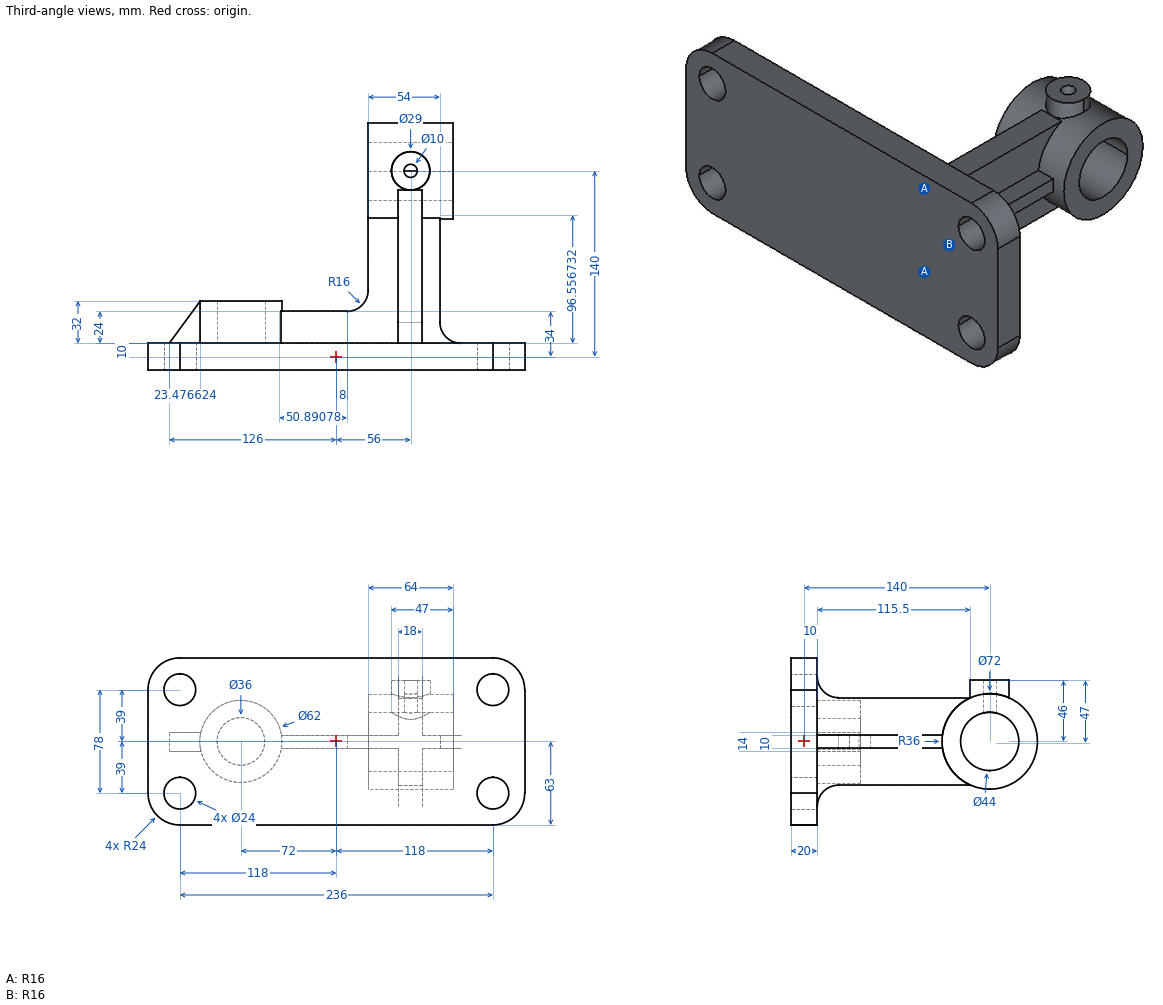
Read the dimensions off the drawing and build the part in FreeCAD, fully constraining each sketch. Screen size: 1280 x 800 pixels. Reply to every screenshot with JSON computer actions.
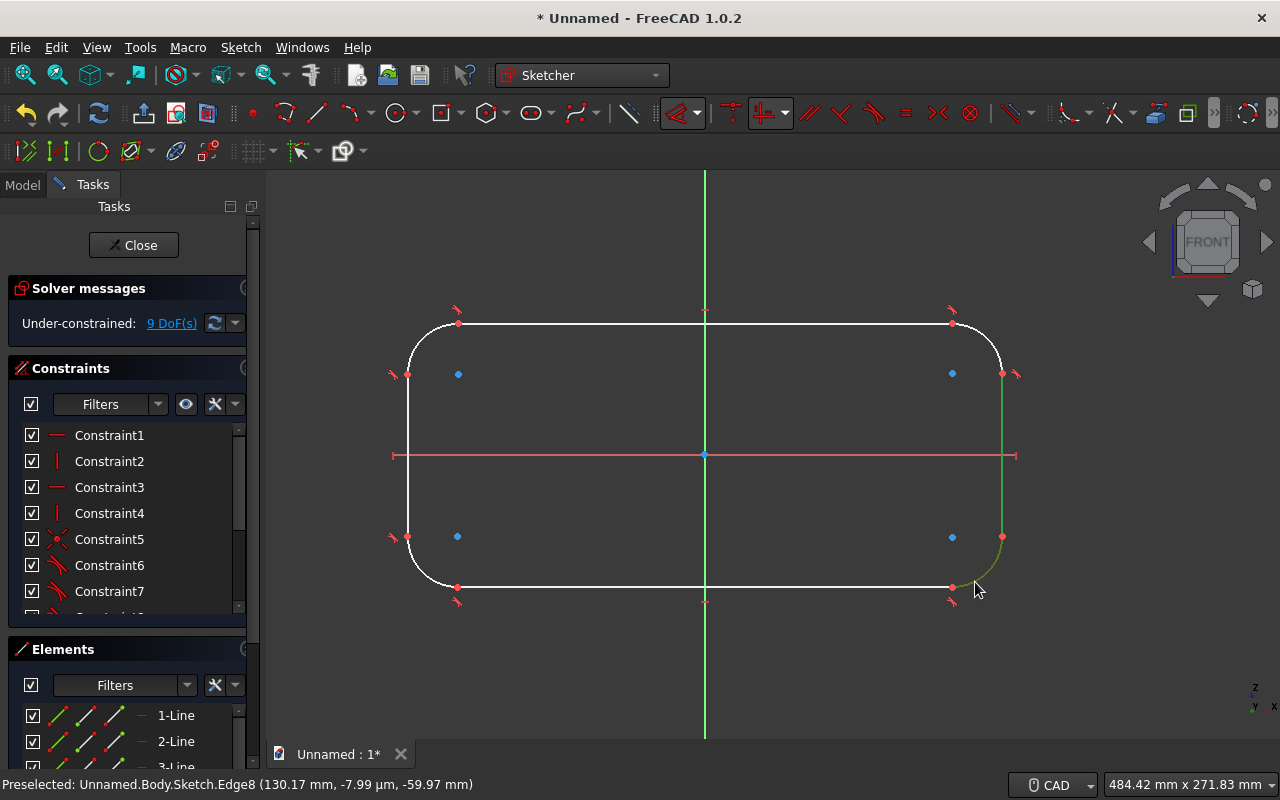
{"action": "left_click", "coordinate": [874, 114]}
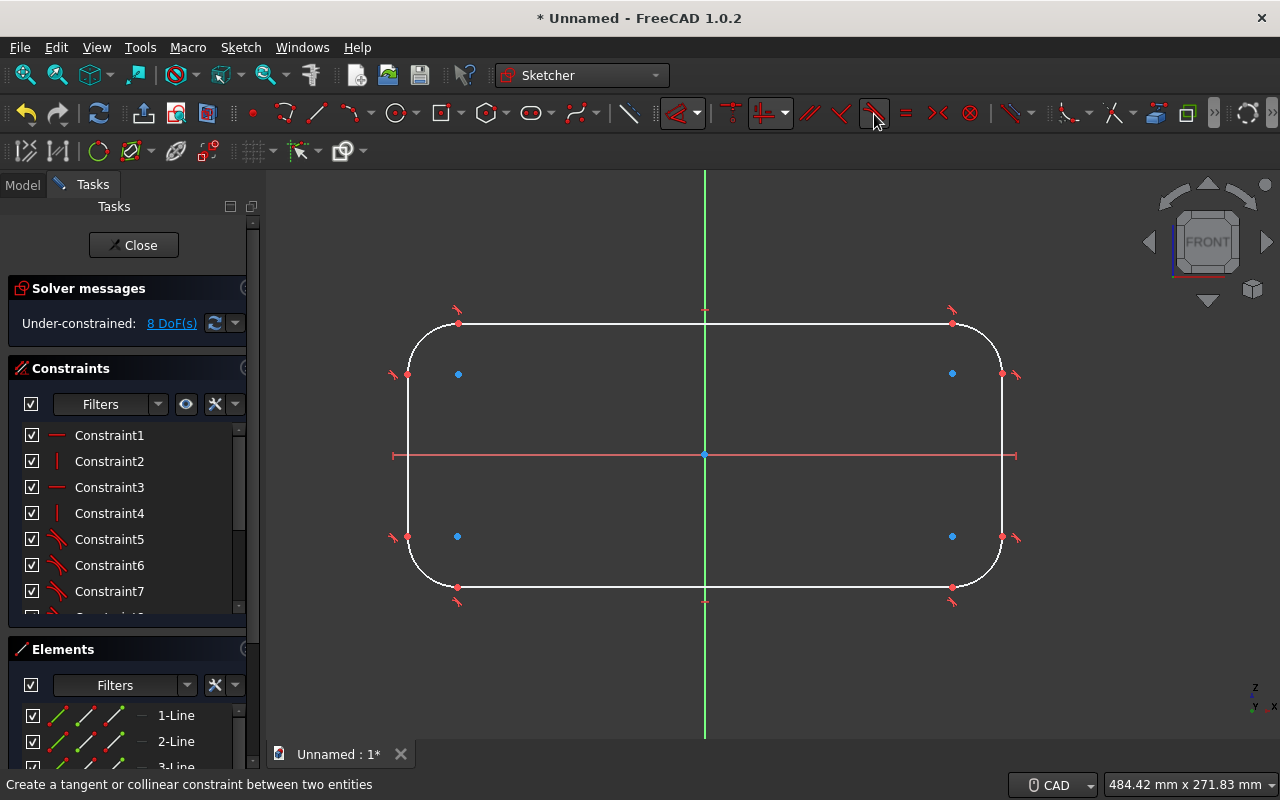
{"action": "left_click", "coordinate": [413, 560]}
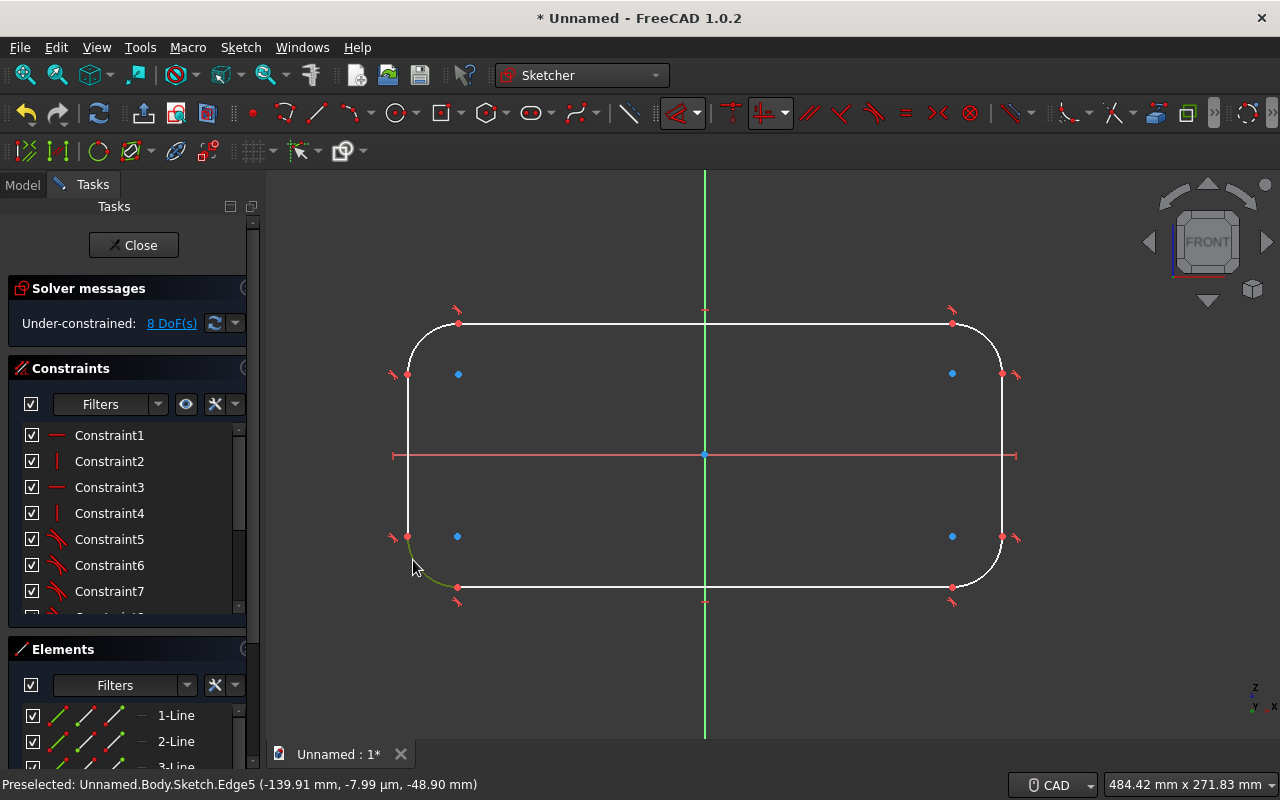
{"action": "left_click", "coordinate": [435, 329]}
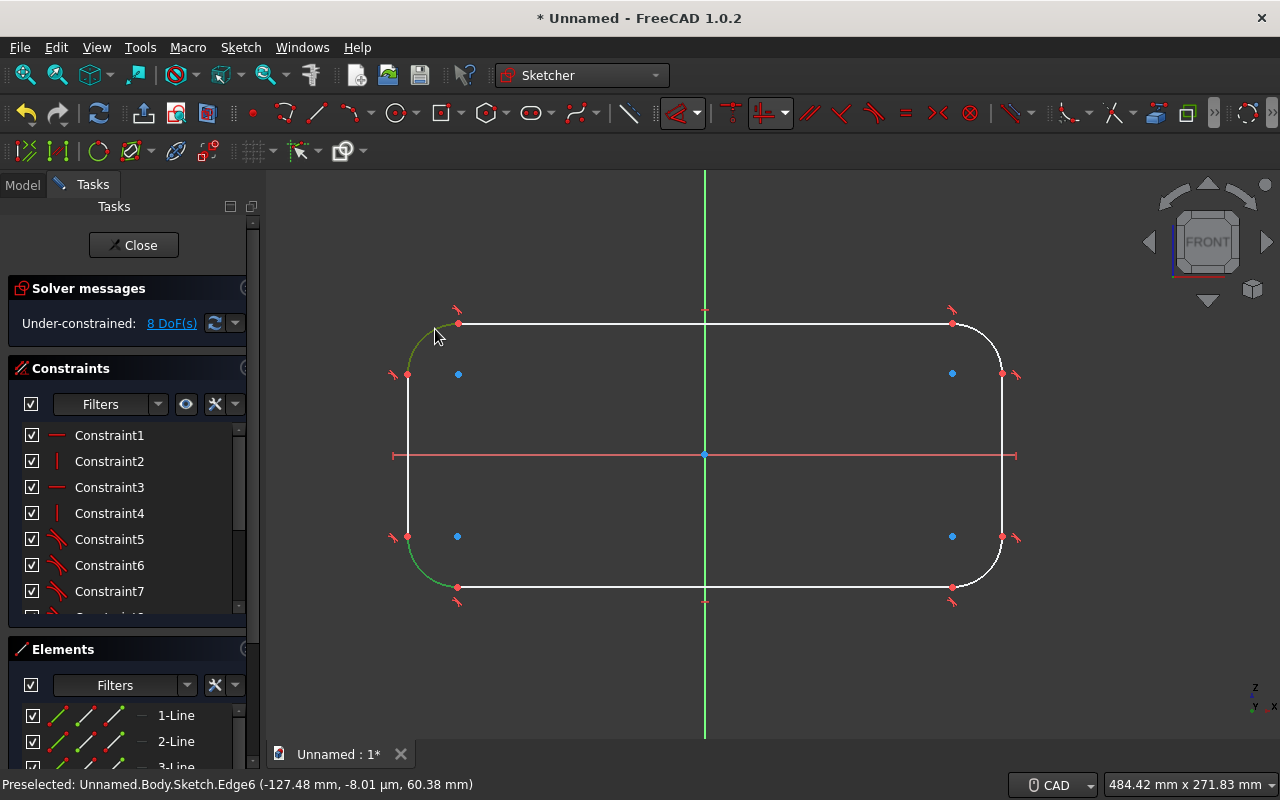
{"action": "left_click", "coordinate": [997, 351]}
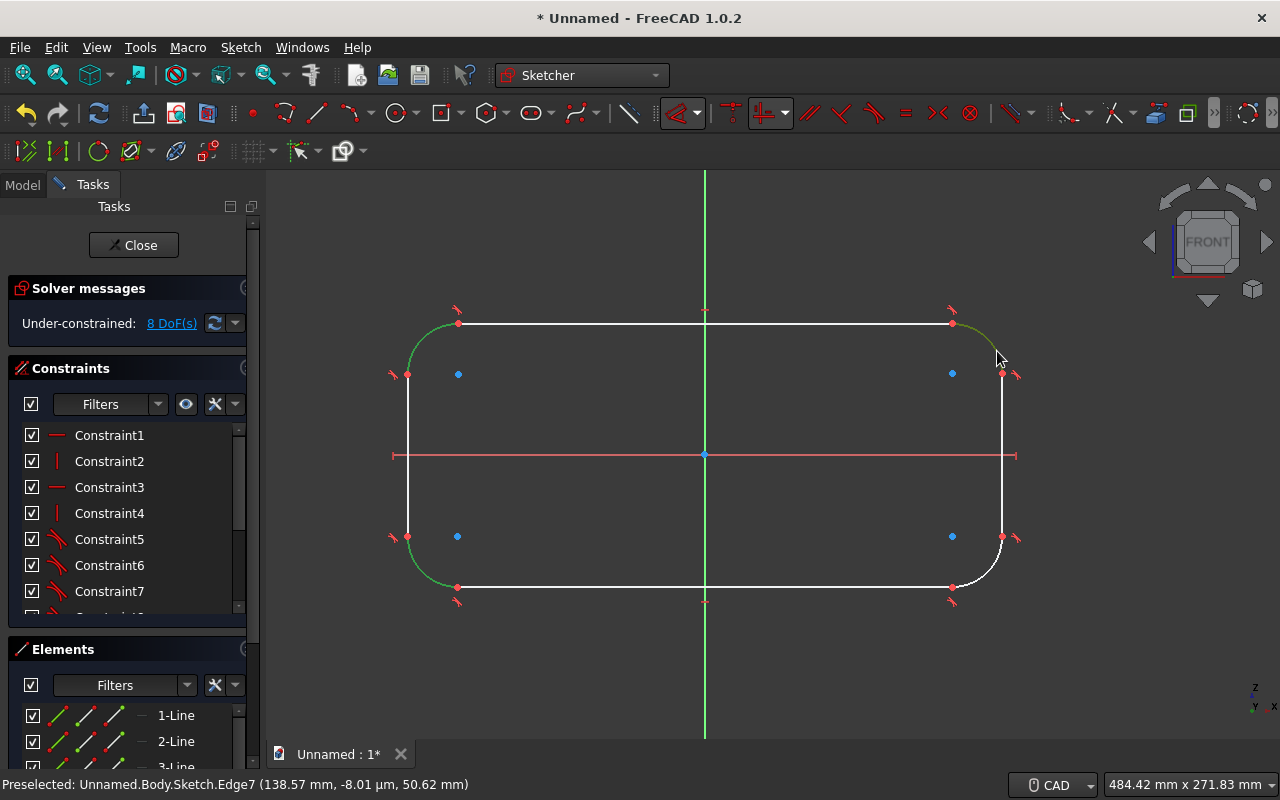
{"action": "left_click", "coordinate": [975, 582]}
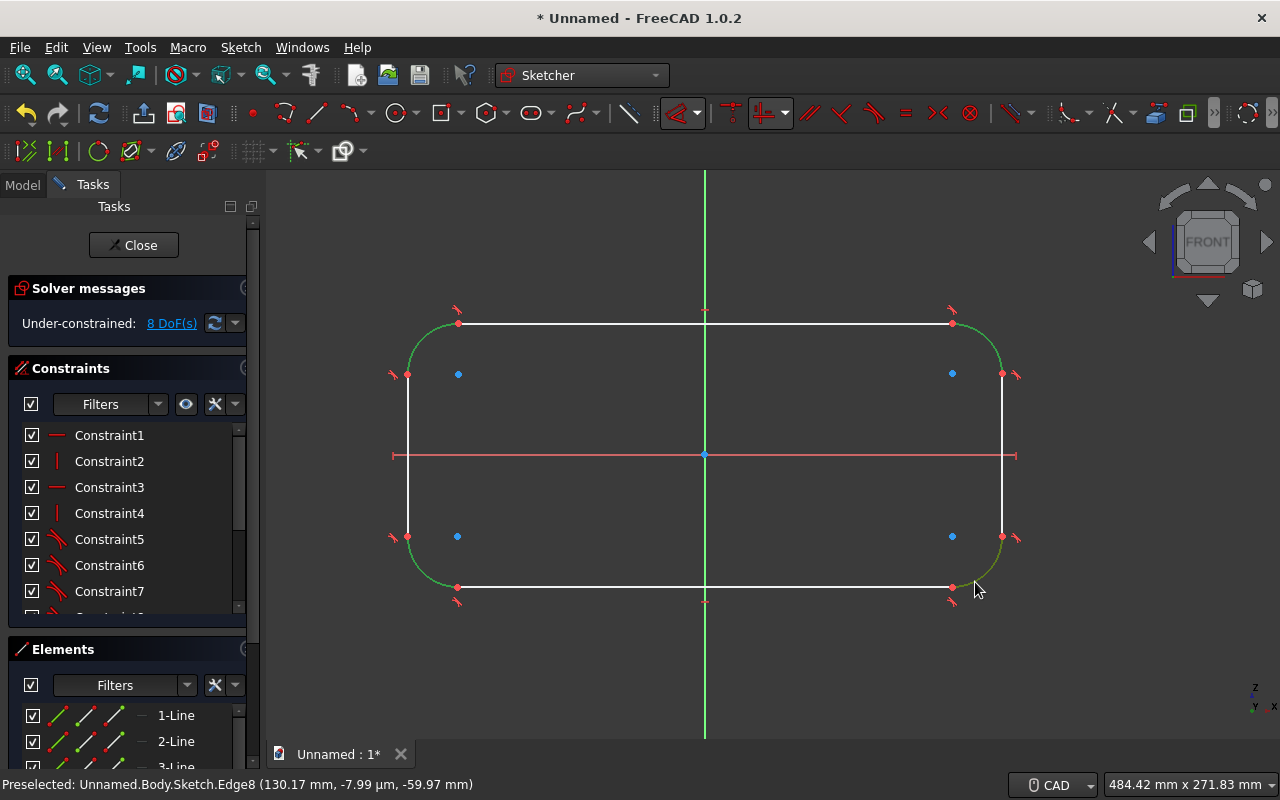
{"action": "left_click", "coordinate": [906, 114]}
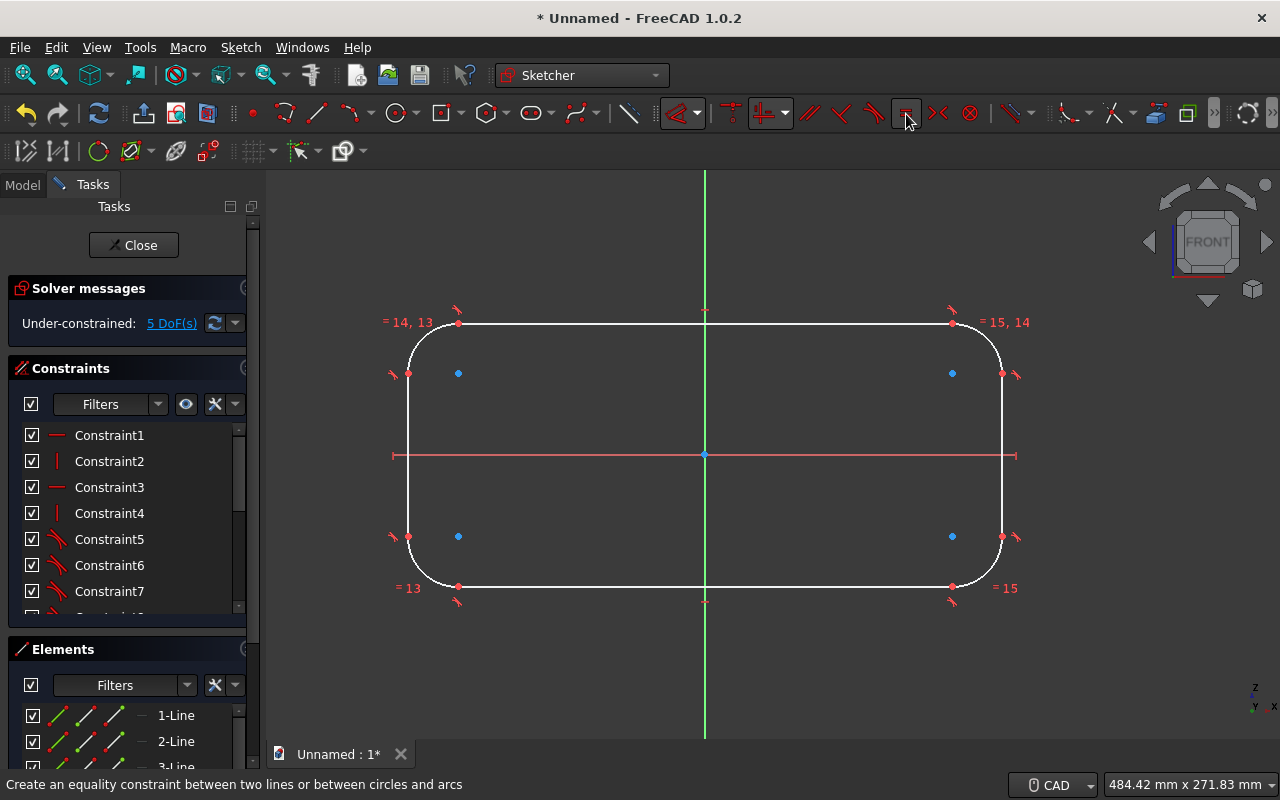
{"action": "left_click", "coordinate": [676, 114]}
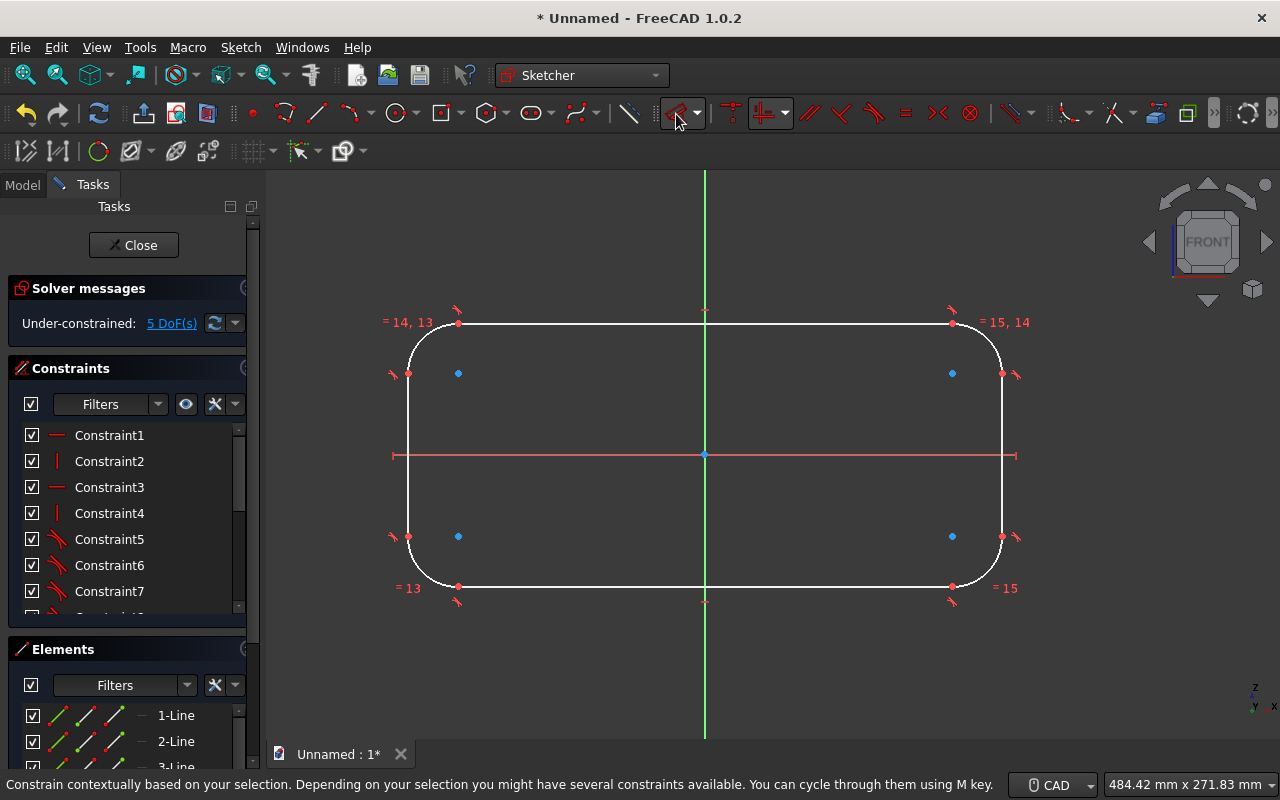
{"action": "left_click", "coordinate": [413, 560]}
{"action": "left_click", "coordinate": [385, 575]}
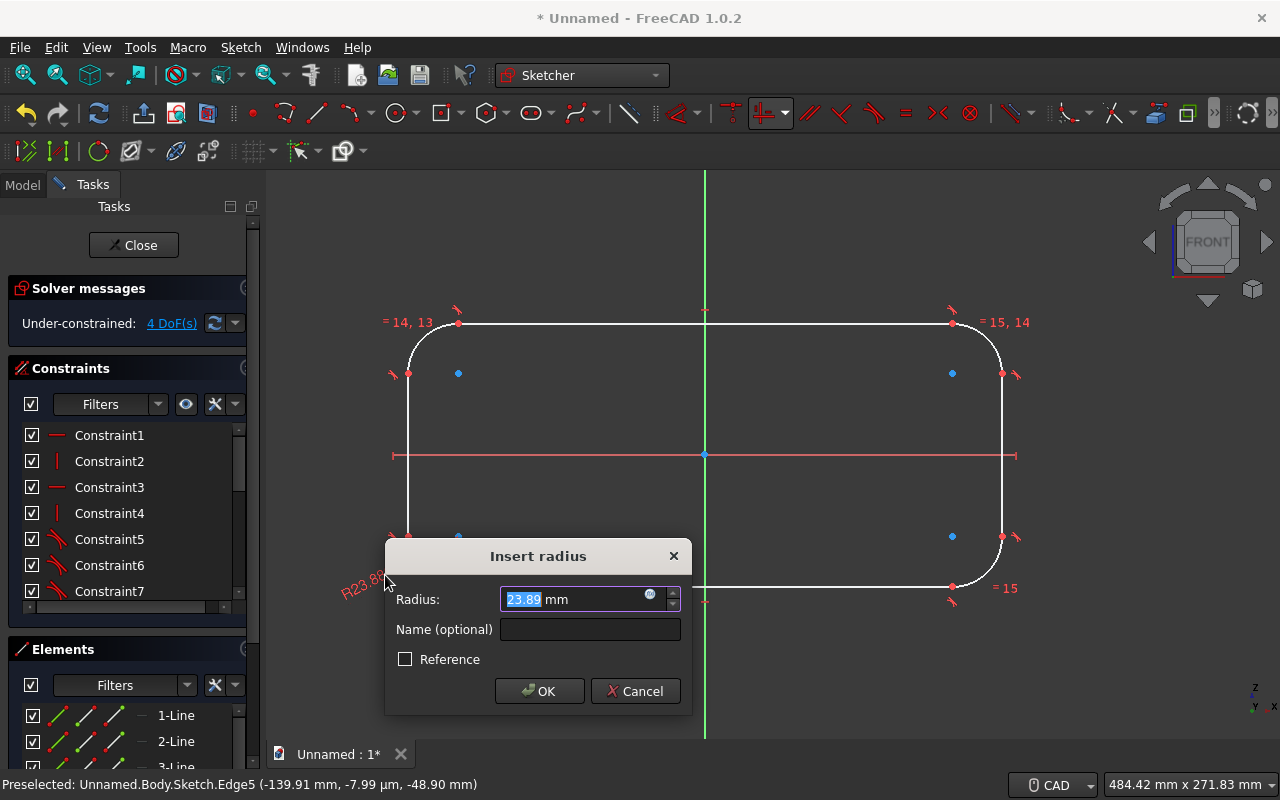
{"action": "type", "text": "24"}
{"action": "key", "text": "Return"}